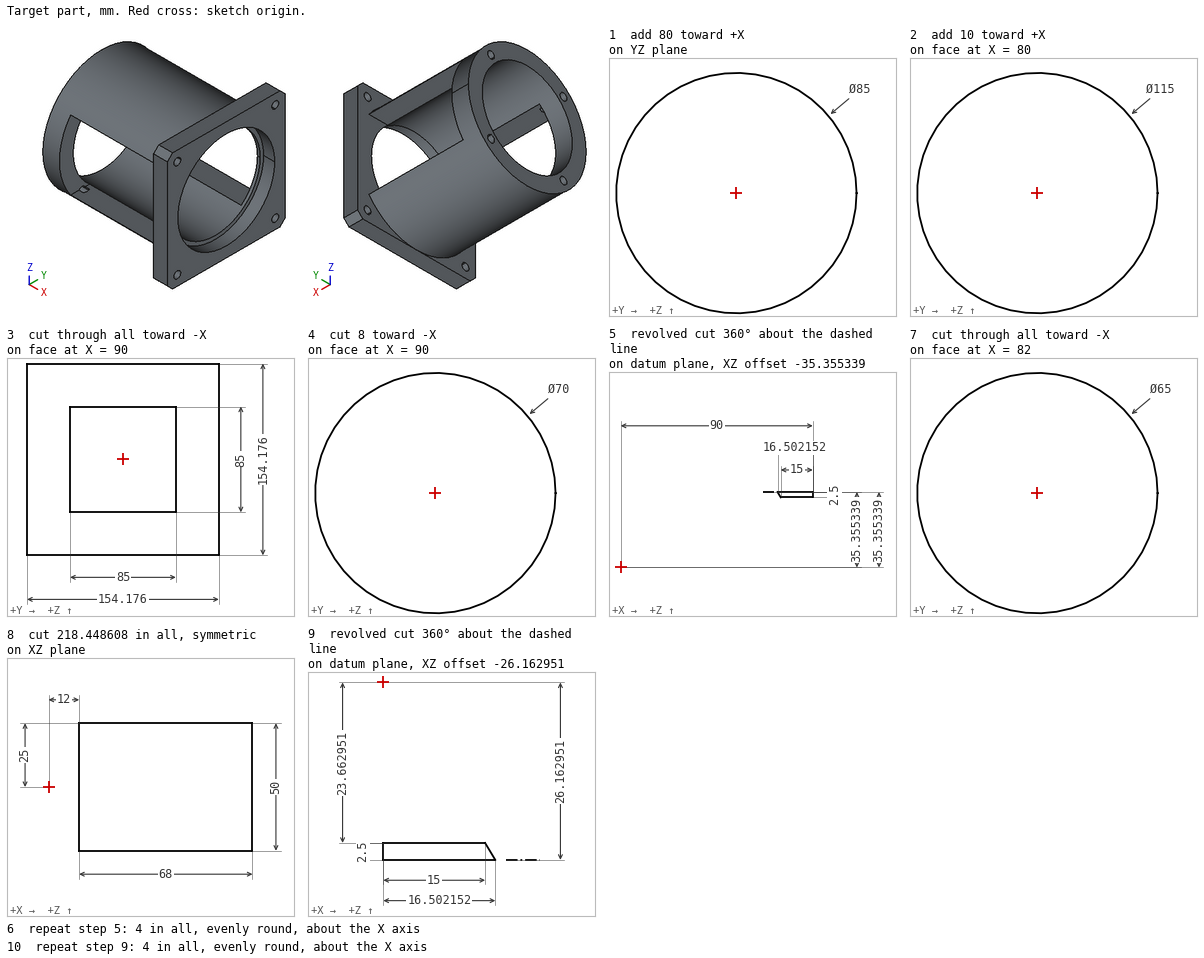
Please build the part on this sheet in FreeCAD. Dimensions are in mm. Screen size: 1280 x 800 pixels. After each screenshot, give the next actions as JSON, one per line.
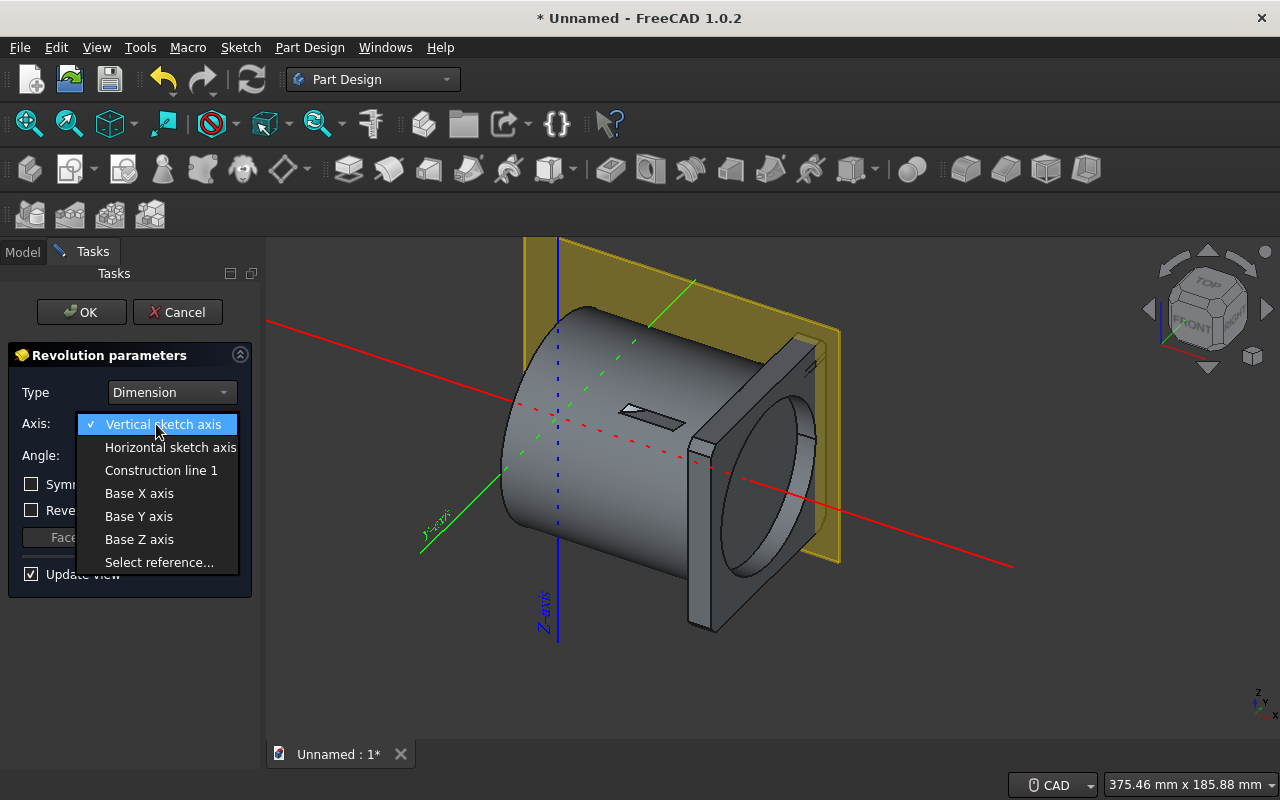
{"action": "left_click", "coordinate": [156, 470]}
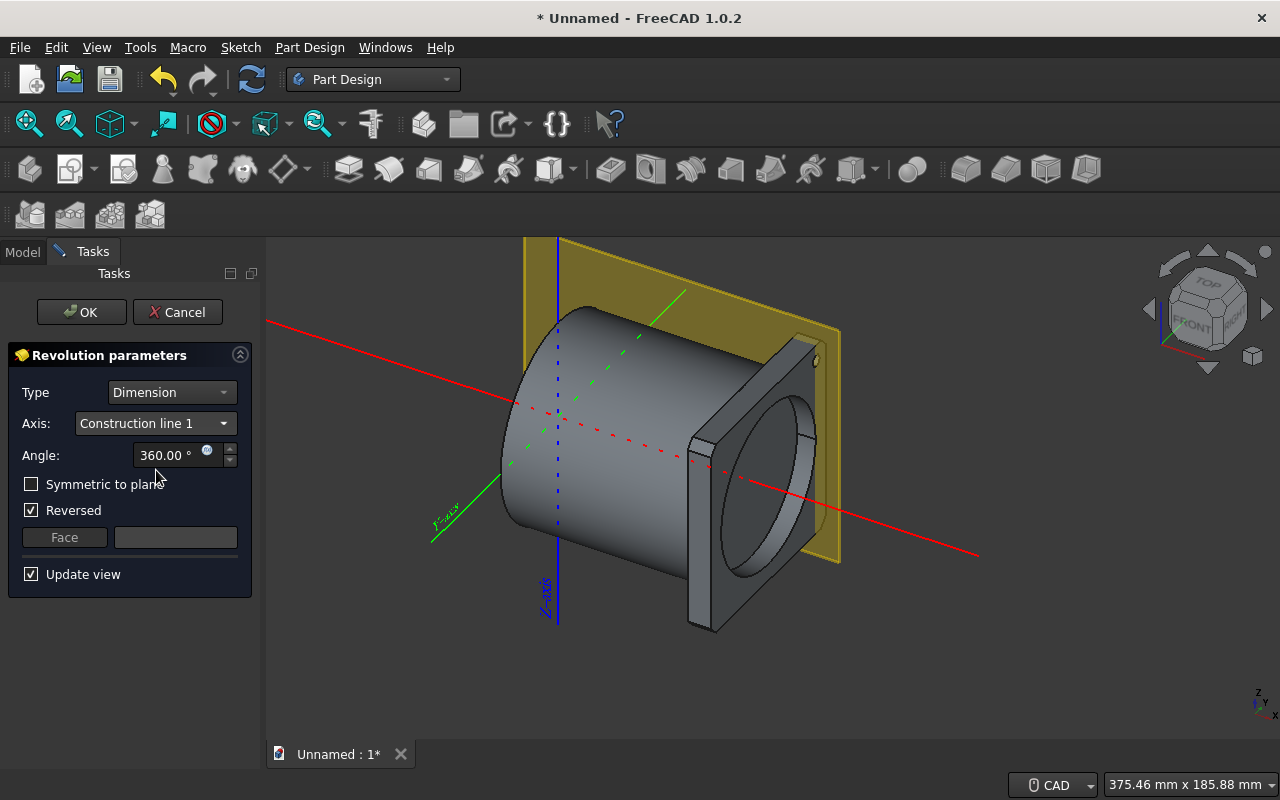
{"action": "left_click", "coordinate": [82, 312]}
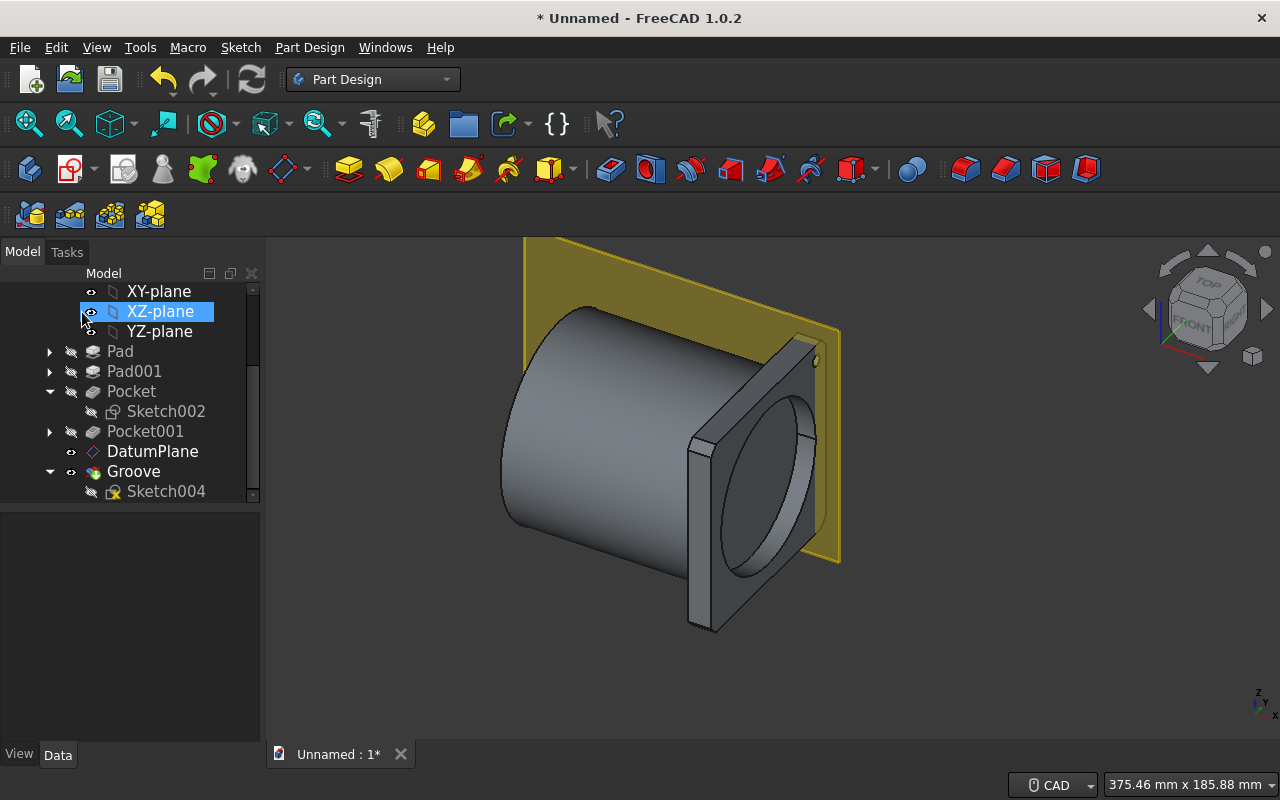
{"action": "left_click", "coordinate": [116, 452]}
{"action": "key", "text": "space"}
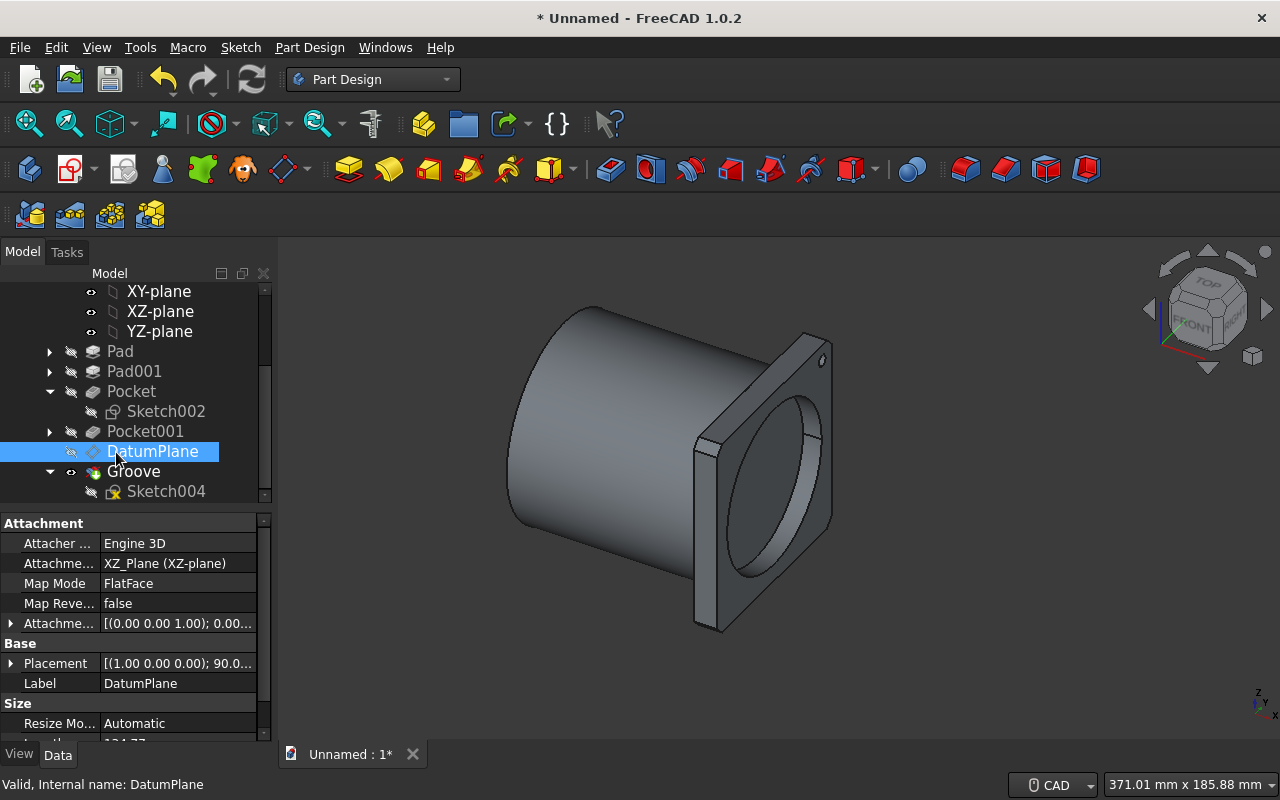
{"action": "left_click", "coordinate": [116, 472]}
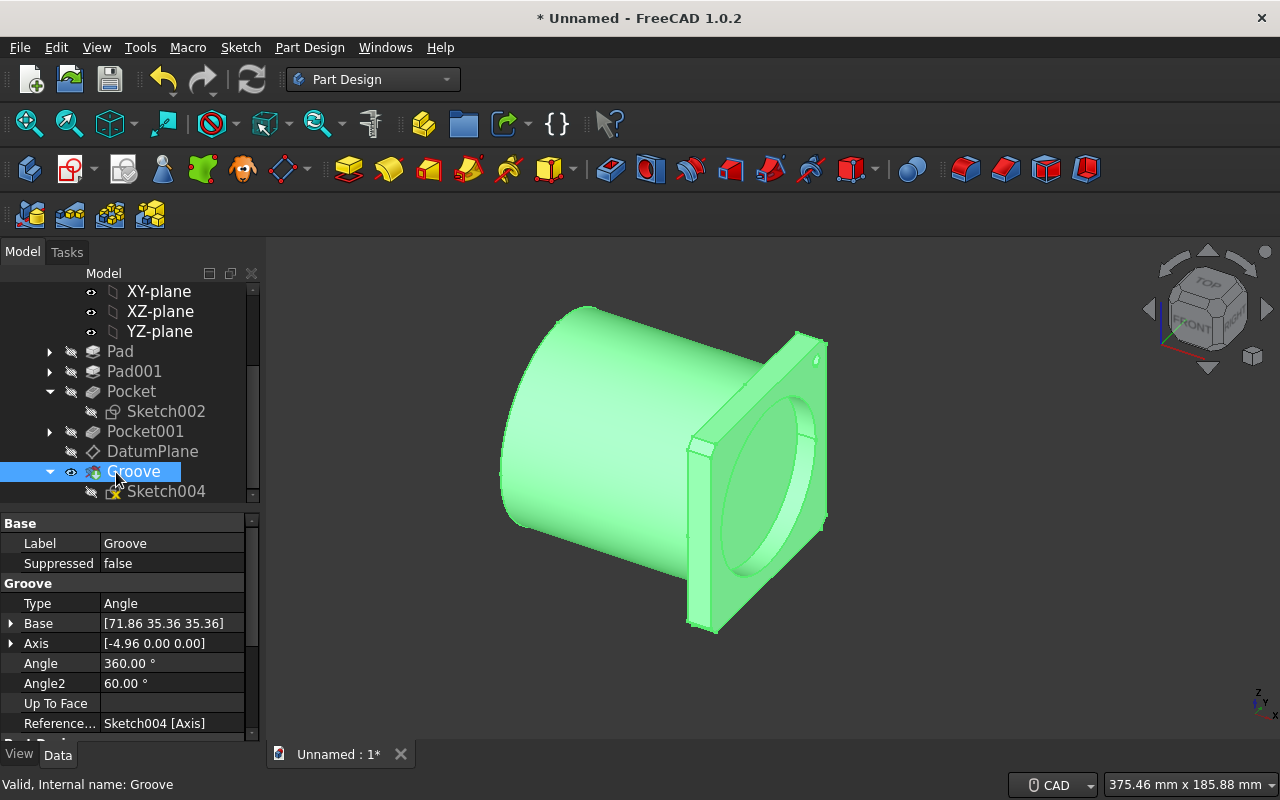
{"action": "left_click", "coordinate": [110, 214]}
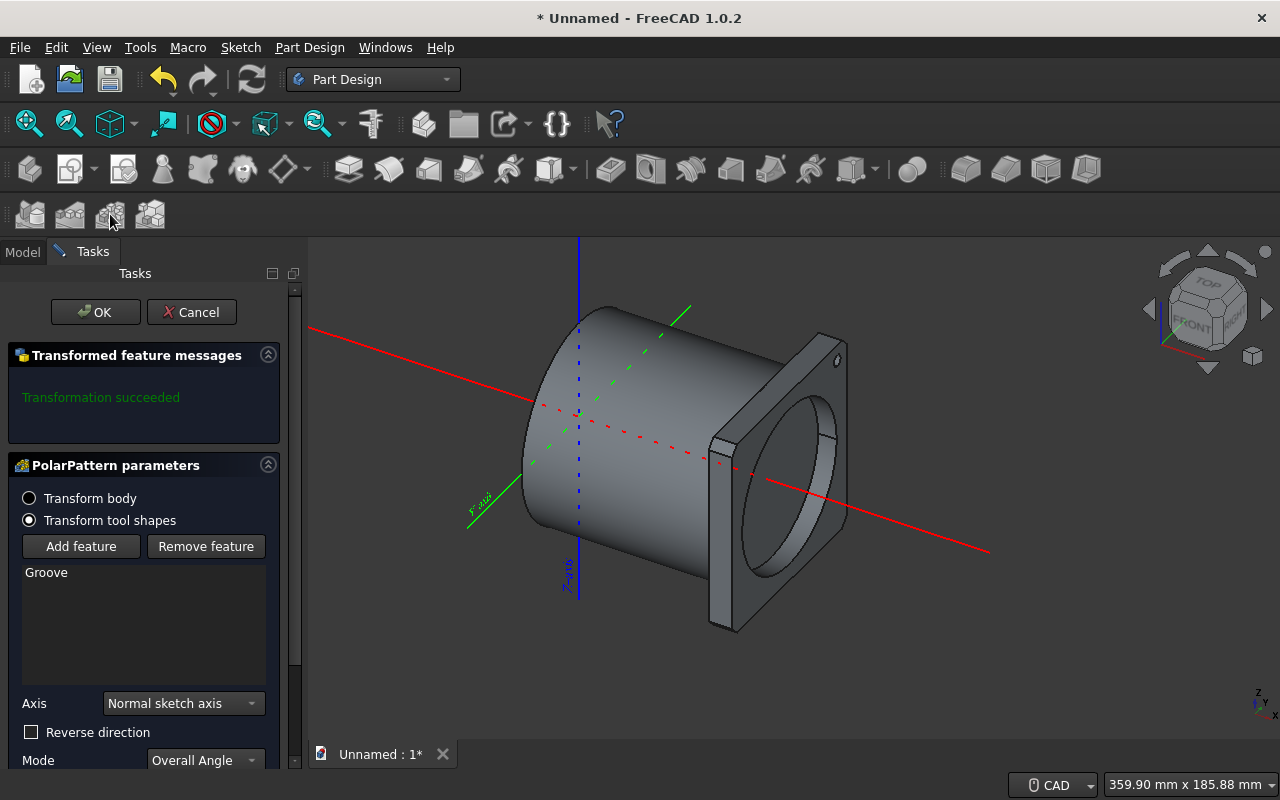
{"action": "left_click", "coordinate": [184, 704]}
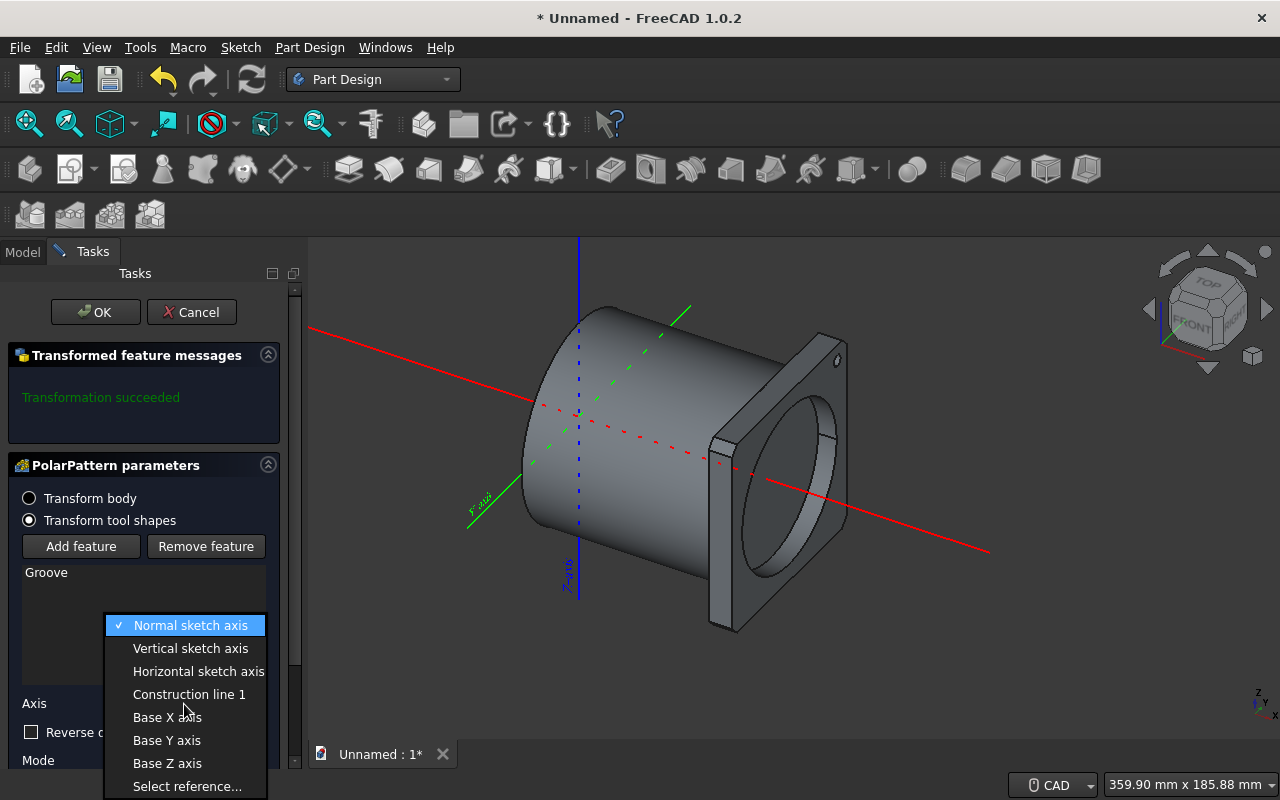
{"action": "left_click", "coordinate": [184, 718]}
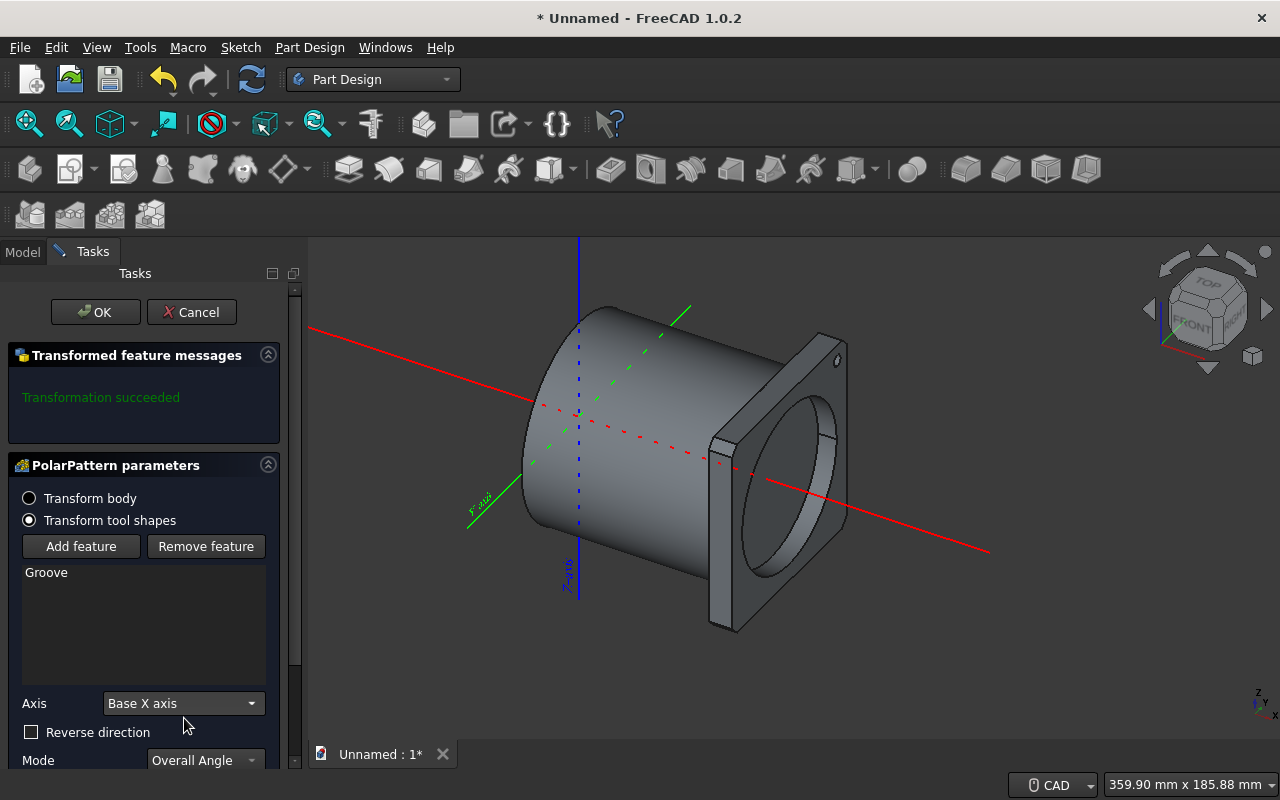
{"action": "scroll", "coordinate": [295, 526], "scroll_direction": "down", "scroll_amount": 3}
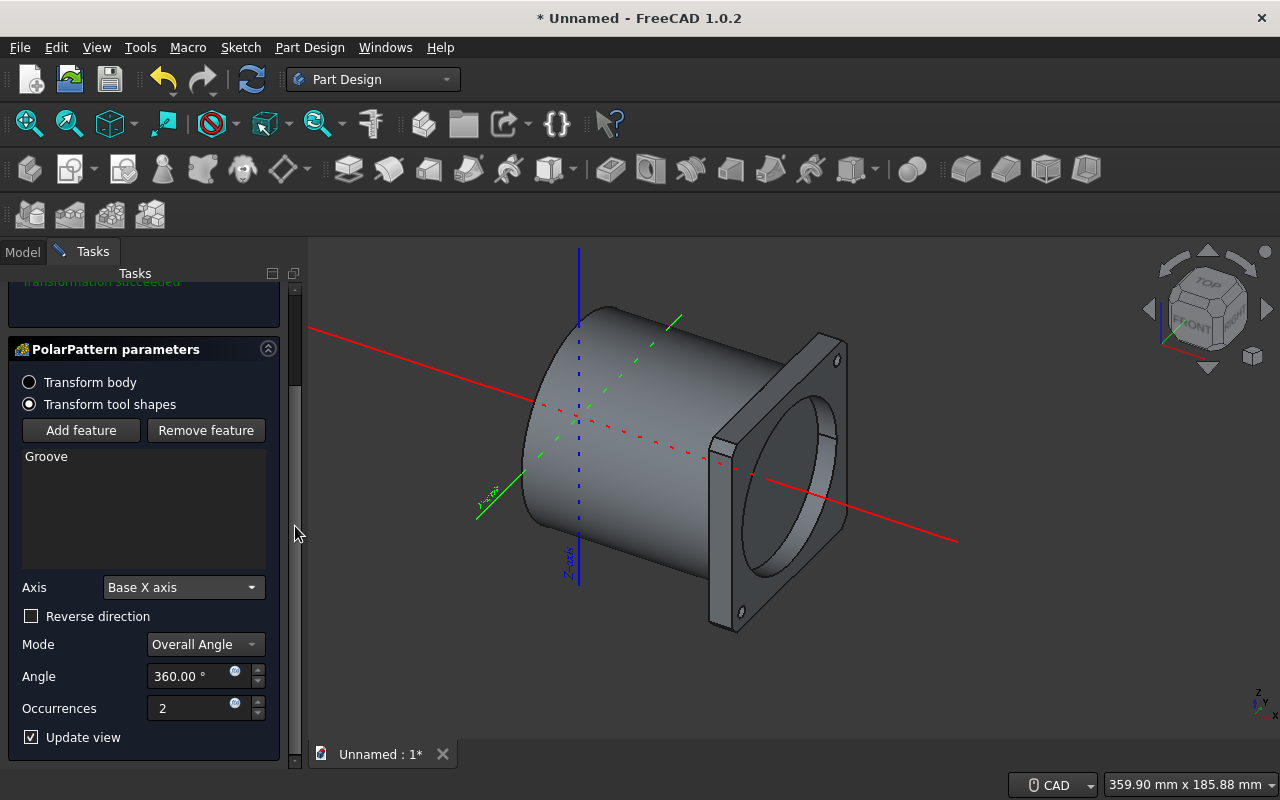
{"action": "triple_click", "coordinate": [198, 708]}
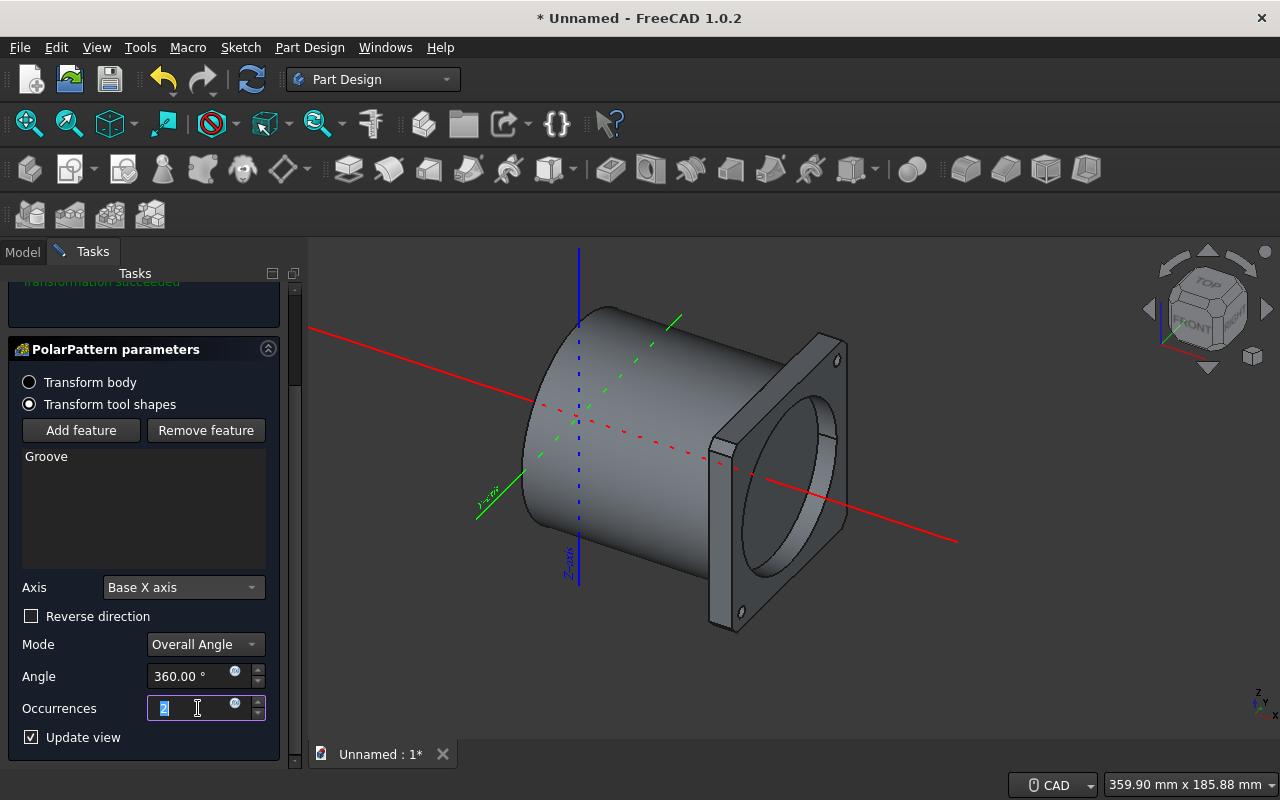
{"action": "type", "text": "4"}
{"action": "key", "text": "Tab"}